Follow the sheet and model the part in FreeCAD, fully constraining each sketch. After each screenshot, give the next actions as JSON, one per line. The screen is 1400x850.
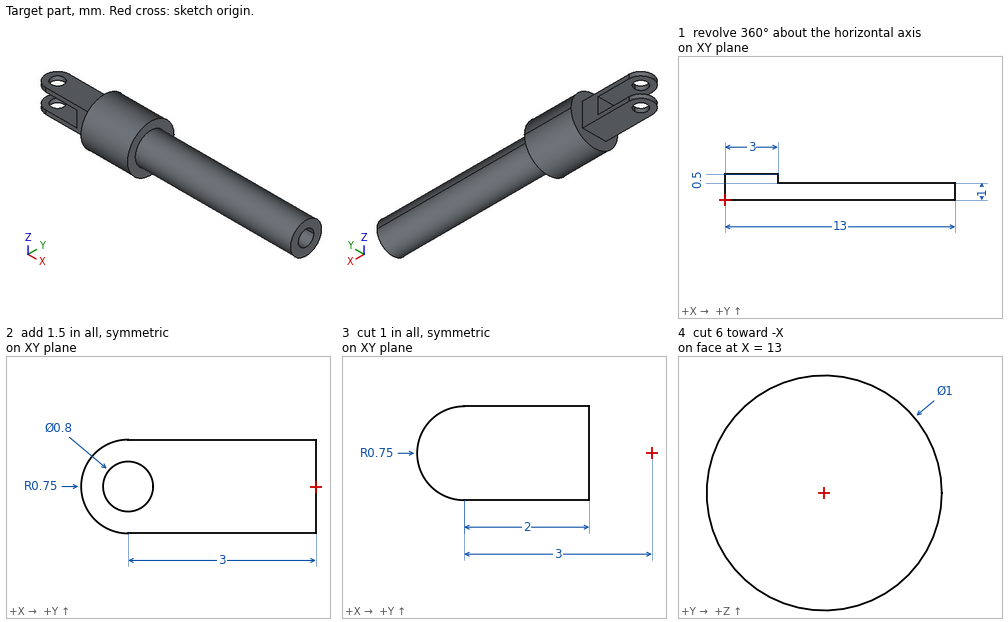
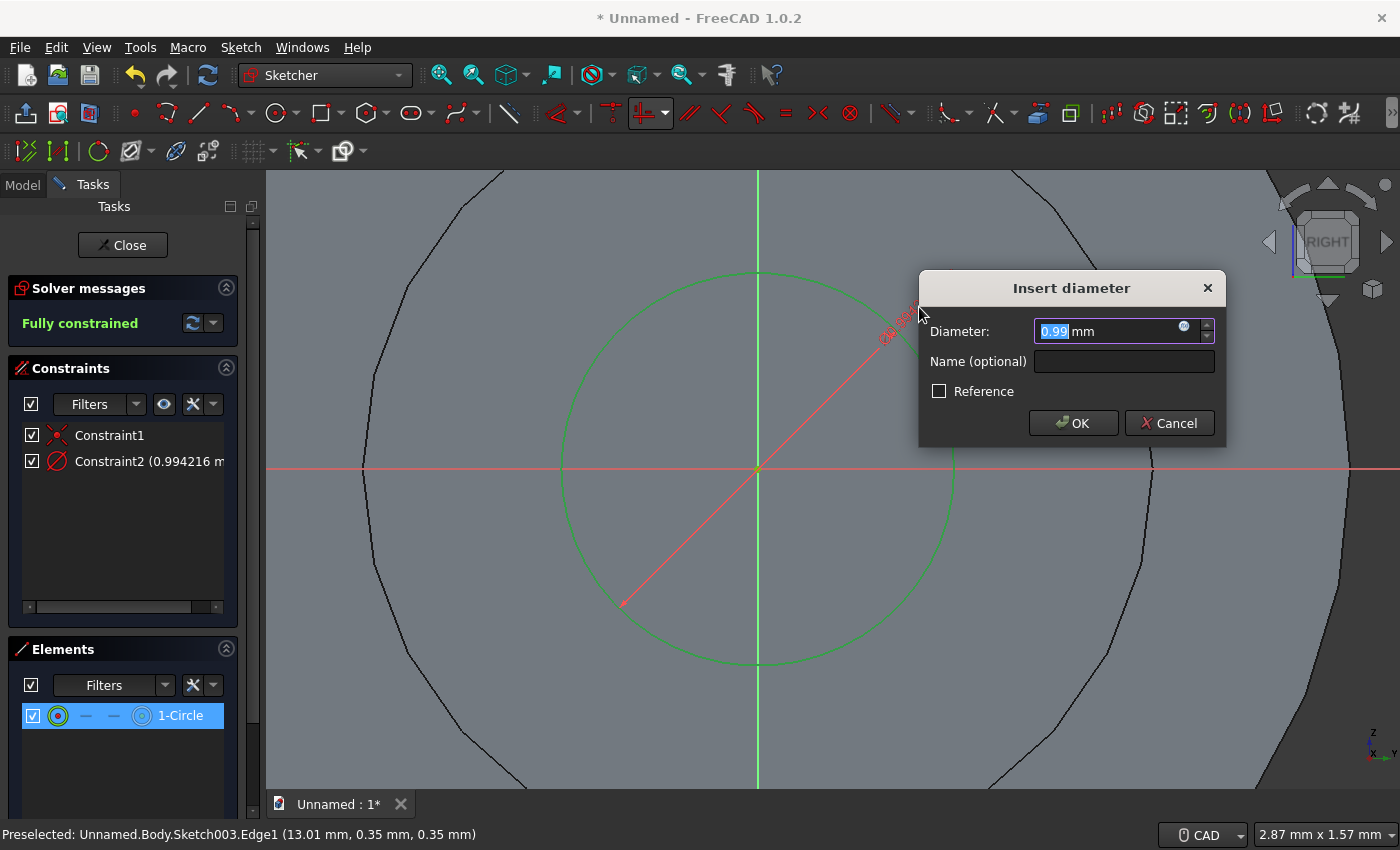
{"action": "type", "text": "1"}
{"action": "key", "text": "Return"}
{"action": "key", "text": "Escape"}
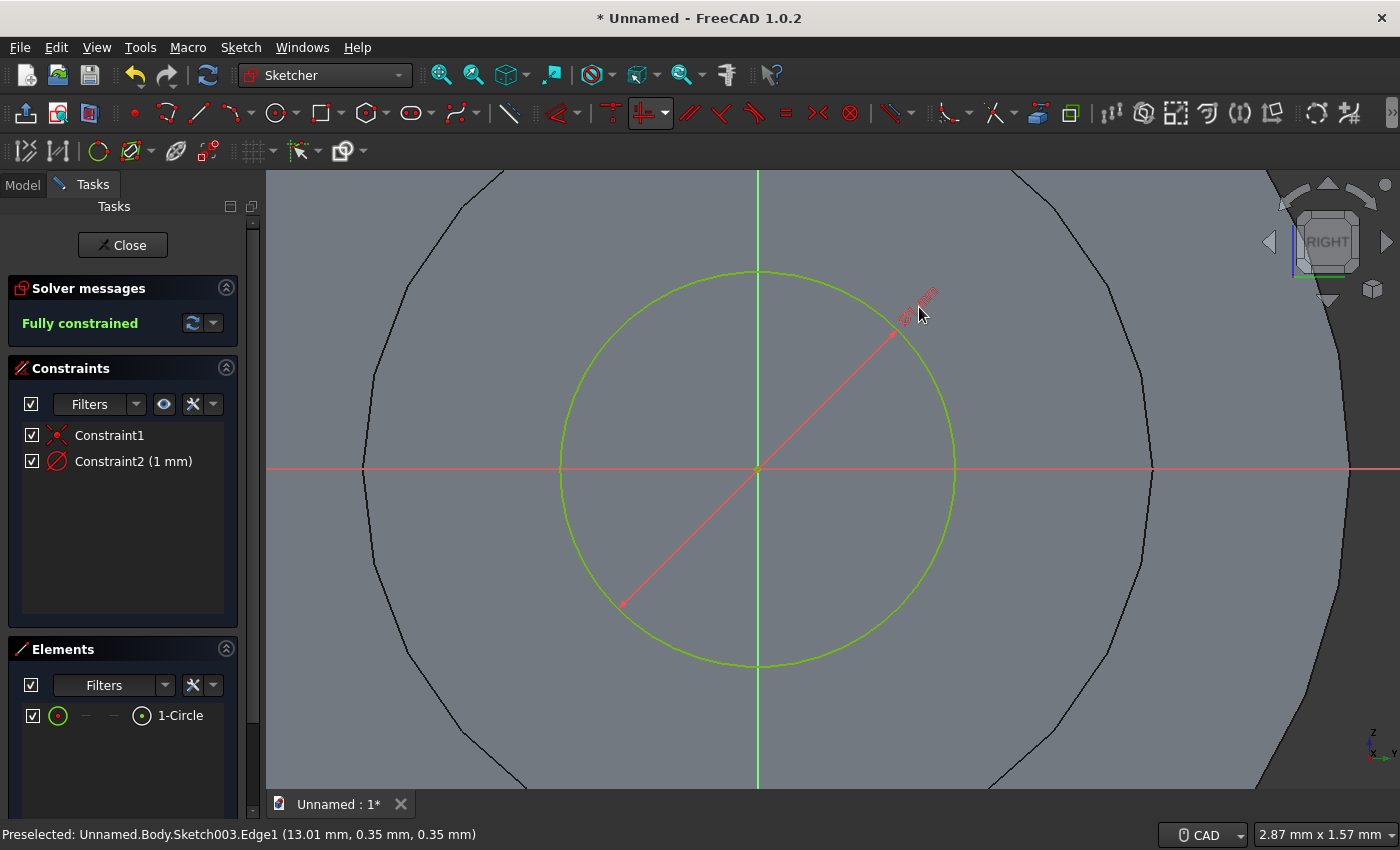
{"action": "left_click", "coordinate": [123, 245]}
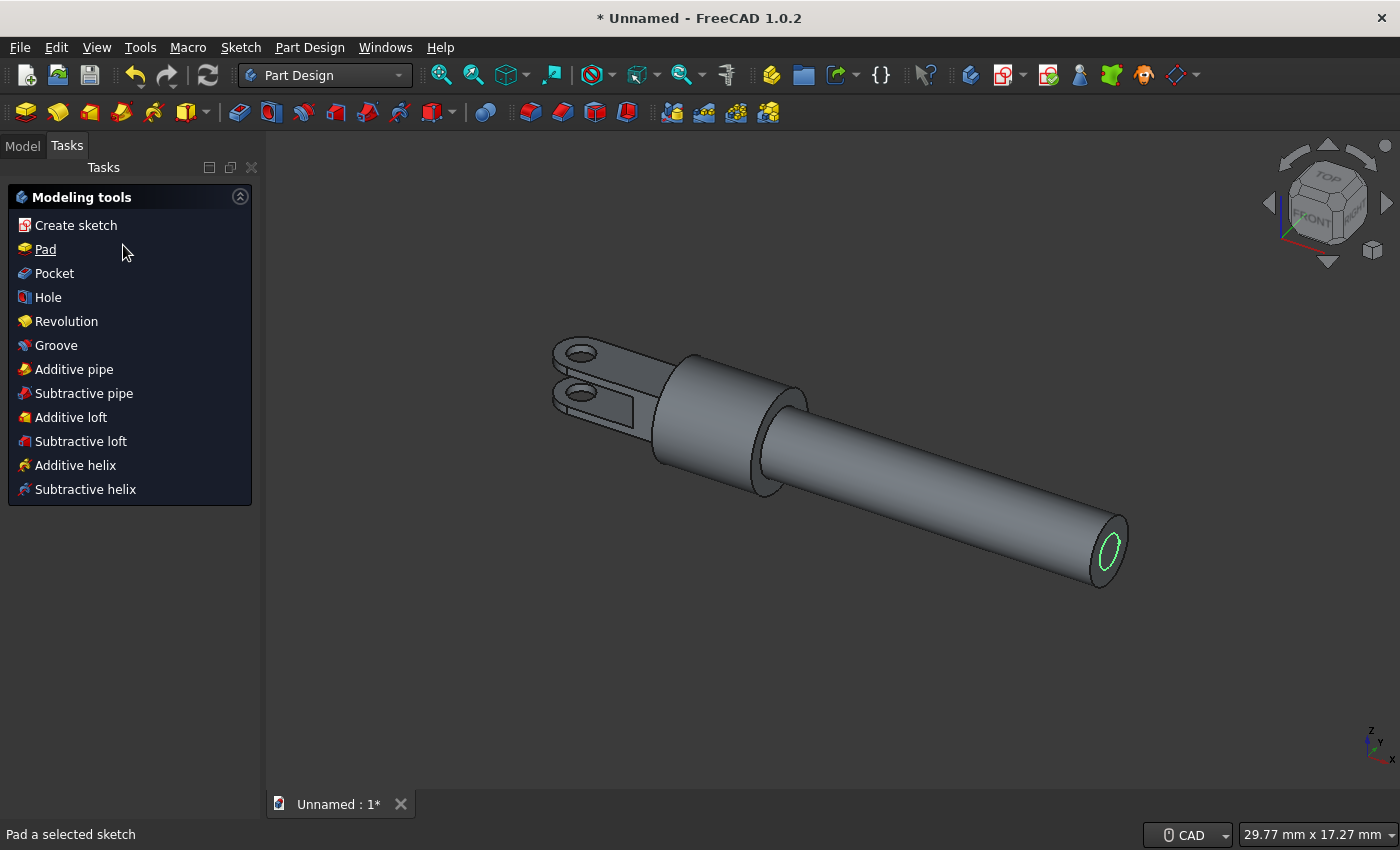
{"action": "left_click", "coordinate": [240, 112]}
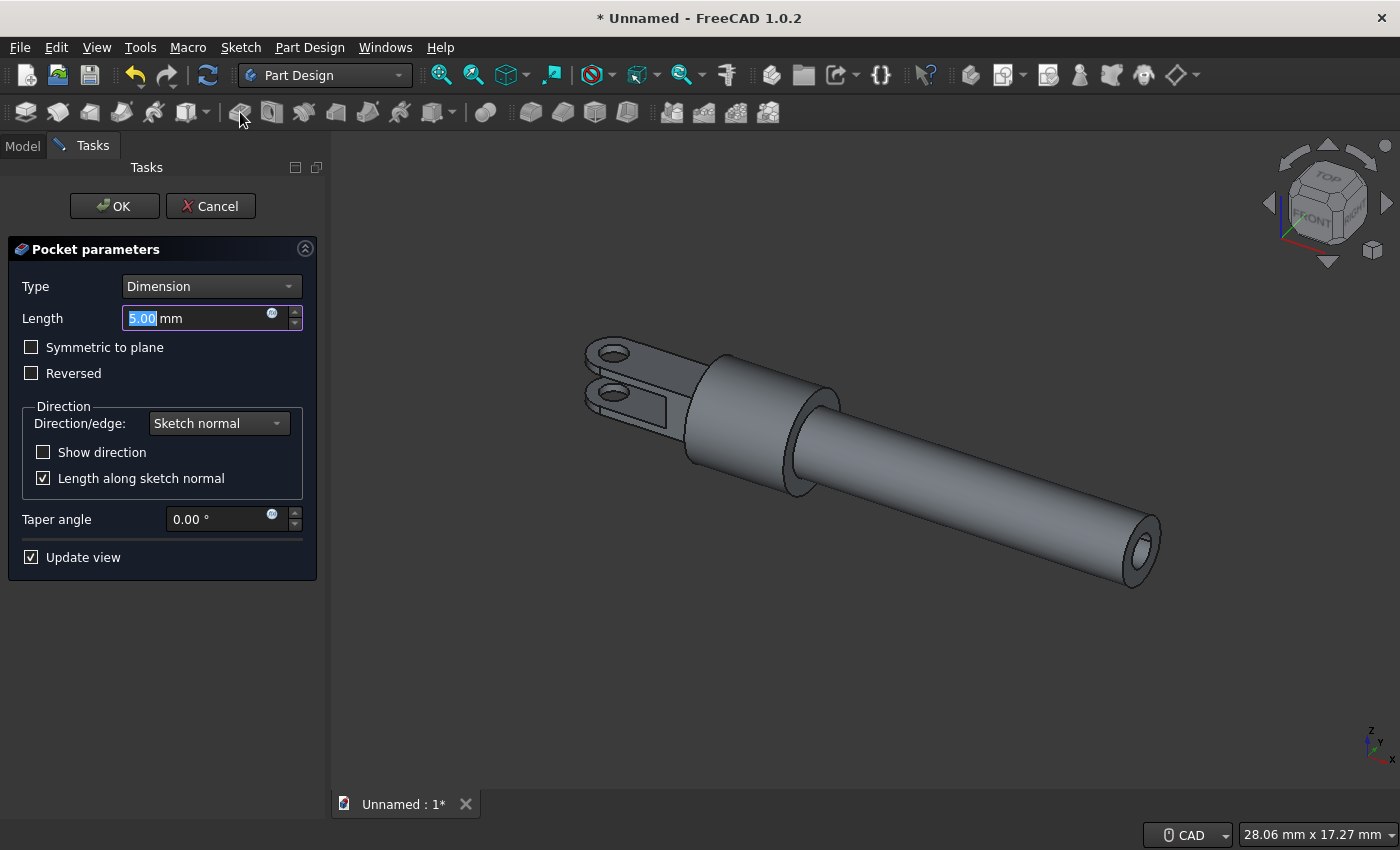
{"action": "type", "text": "6"}
{"action": "key", "text": "Tab"}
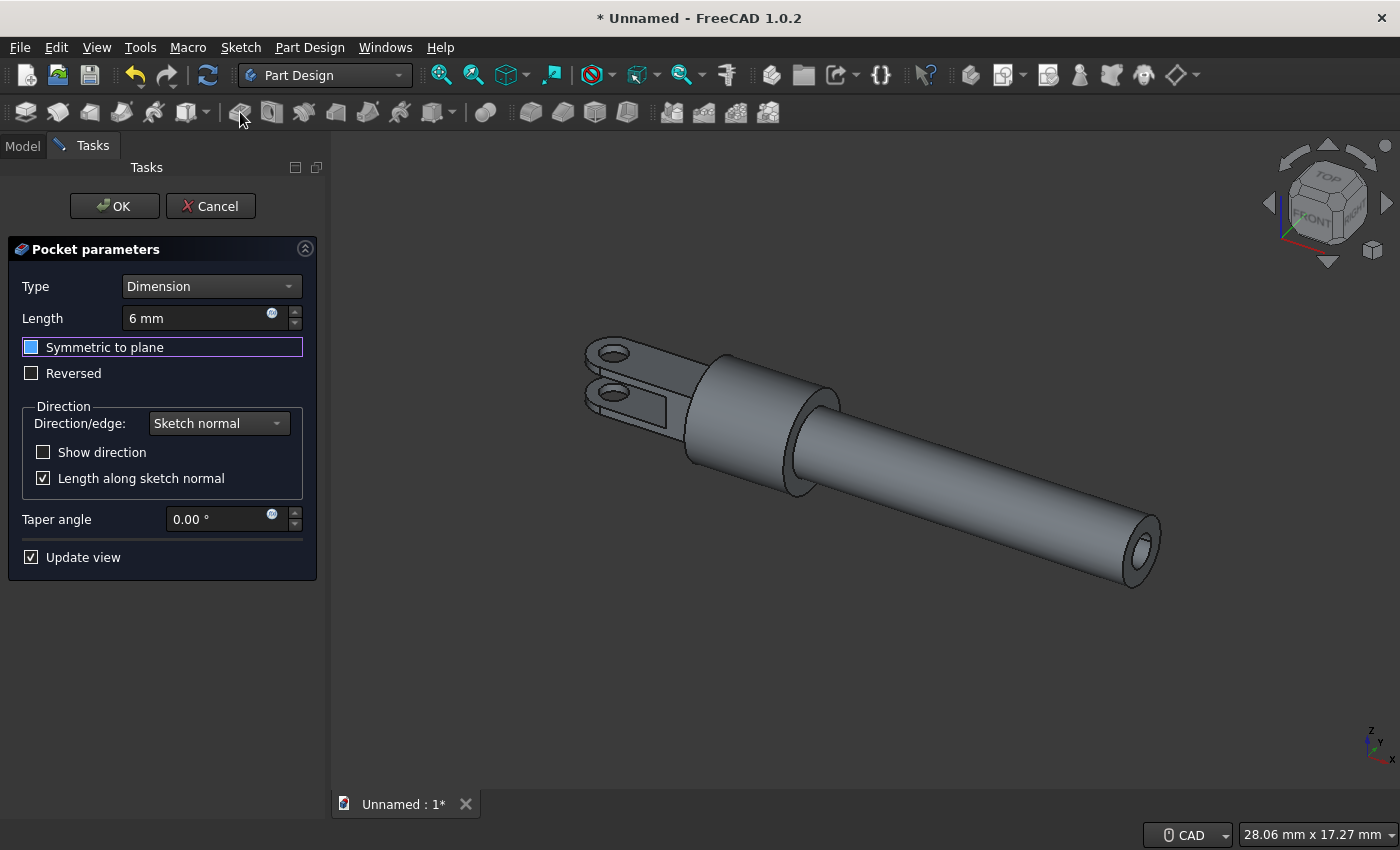
{"action": "left_click", "coordinate": [115, 206]}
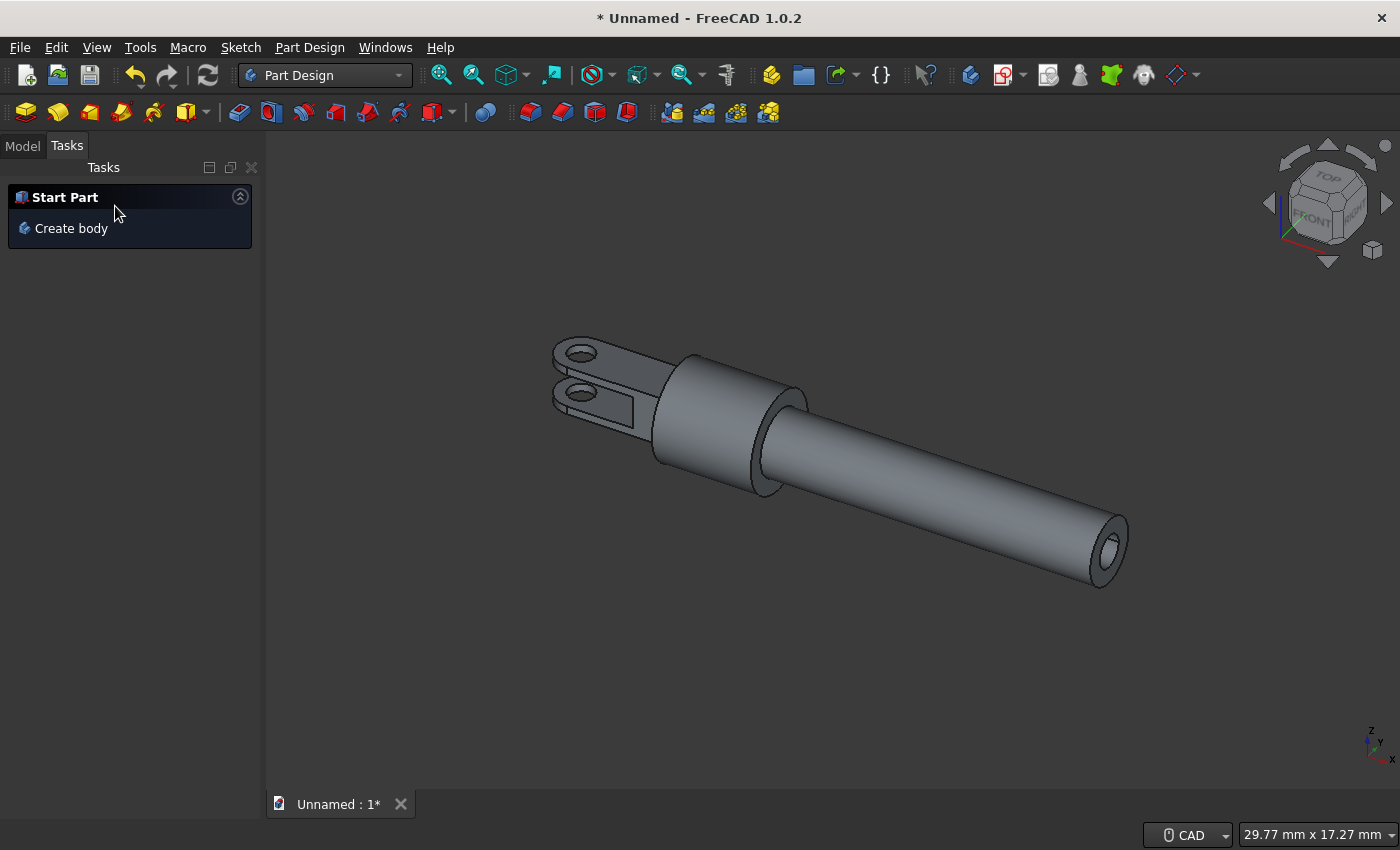
{"action": "key", "text": "0"}